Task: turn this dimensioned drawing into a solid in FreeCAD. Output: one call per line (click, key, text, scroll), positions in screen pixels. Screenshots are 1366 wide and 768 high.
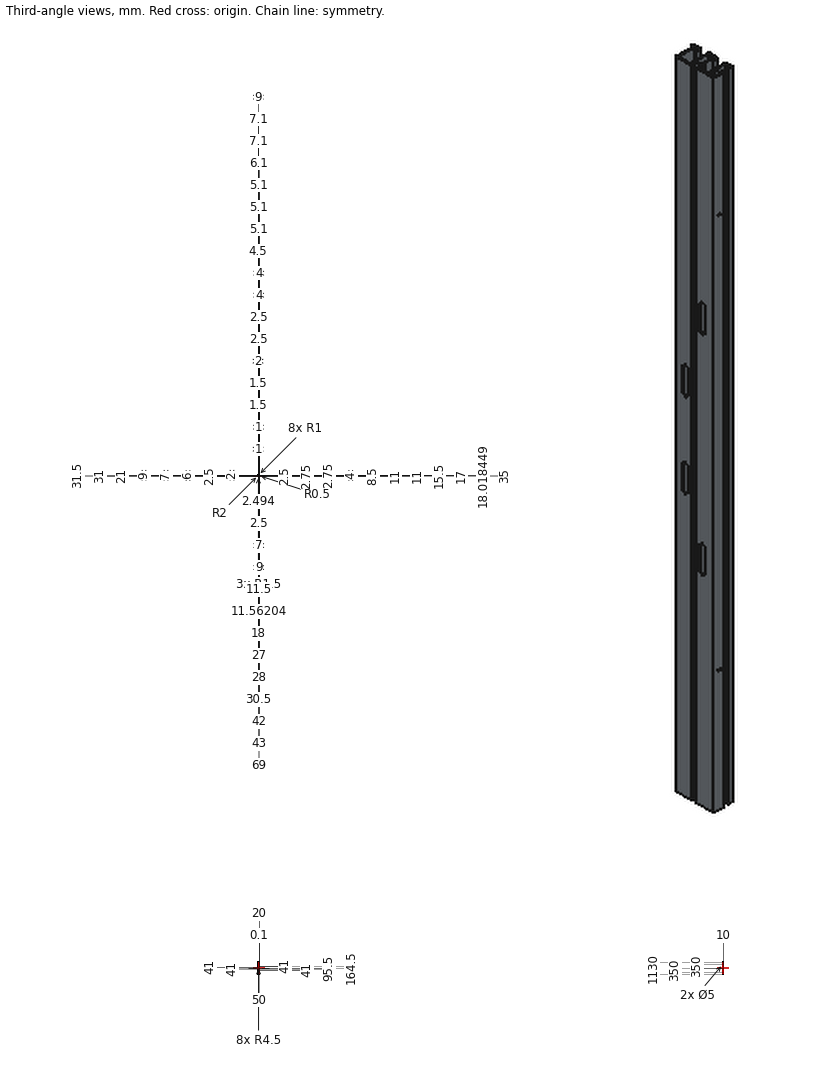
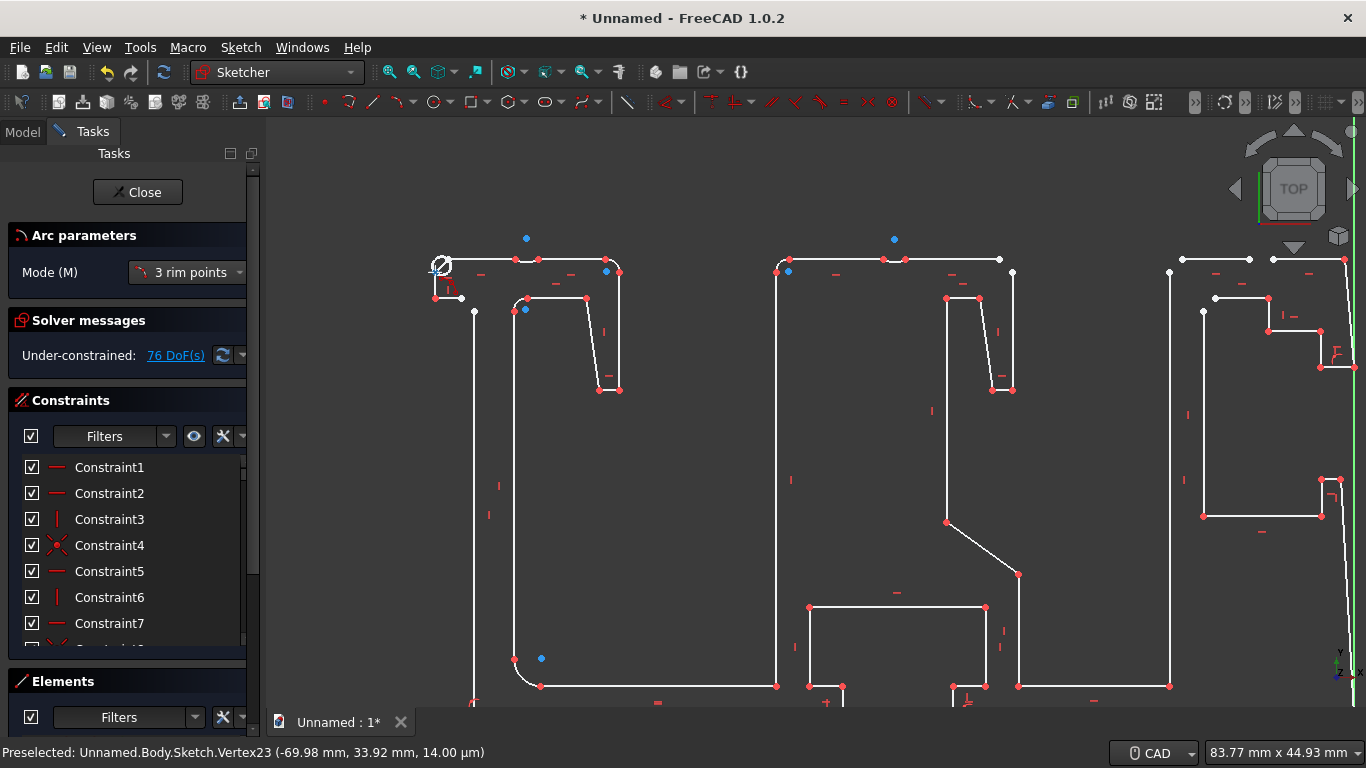
scroll(439, 262, up, 8)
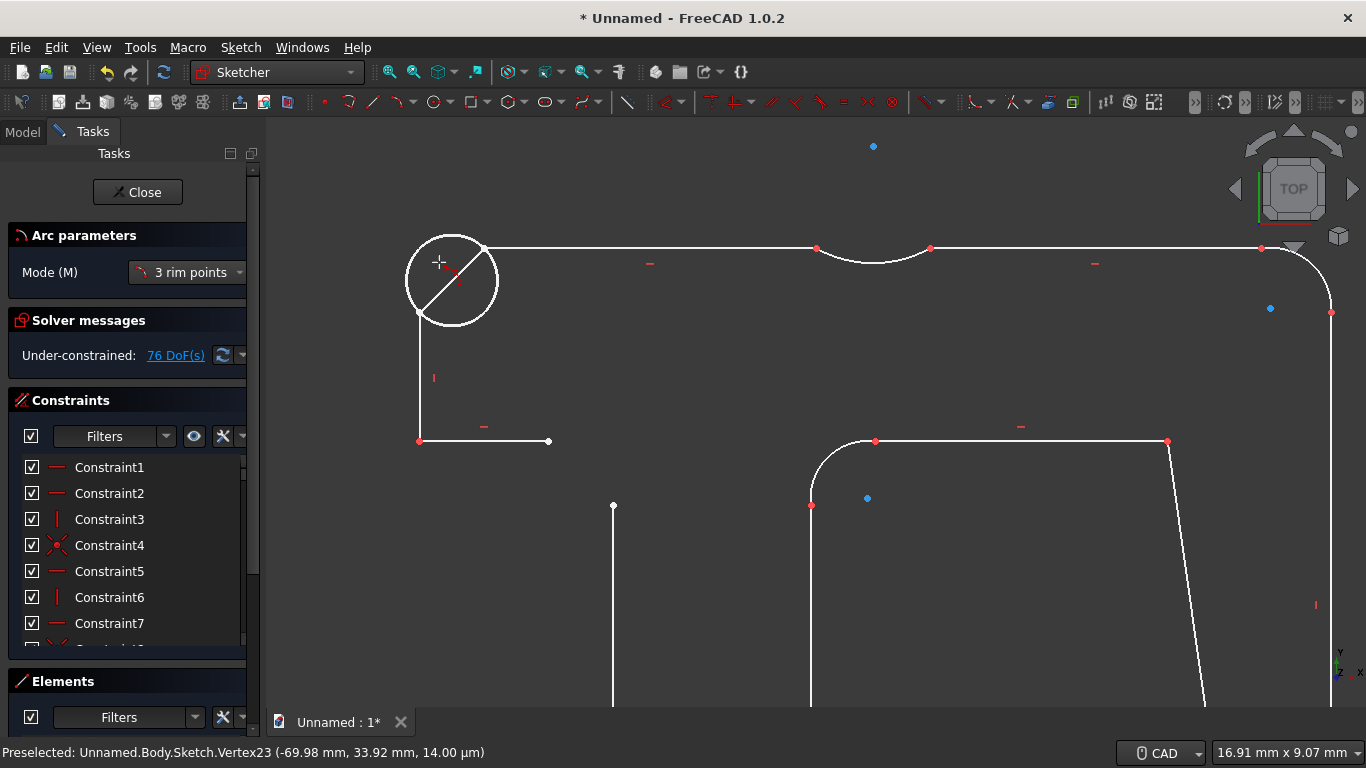
click(438, 261)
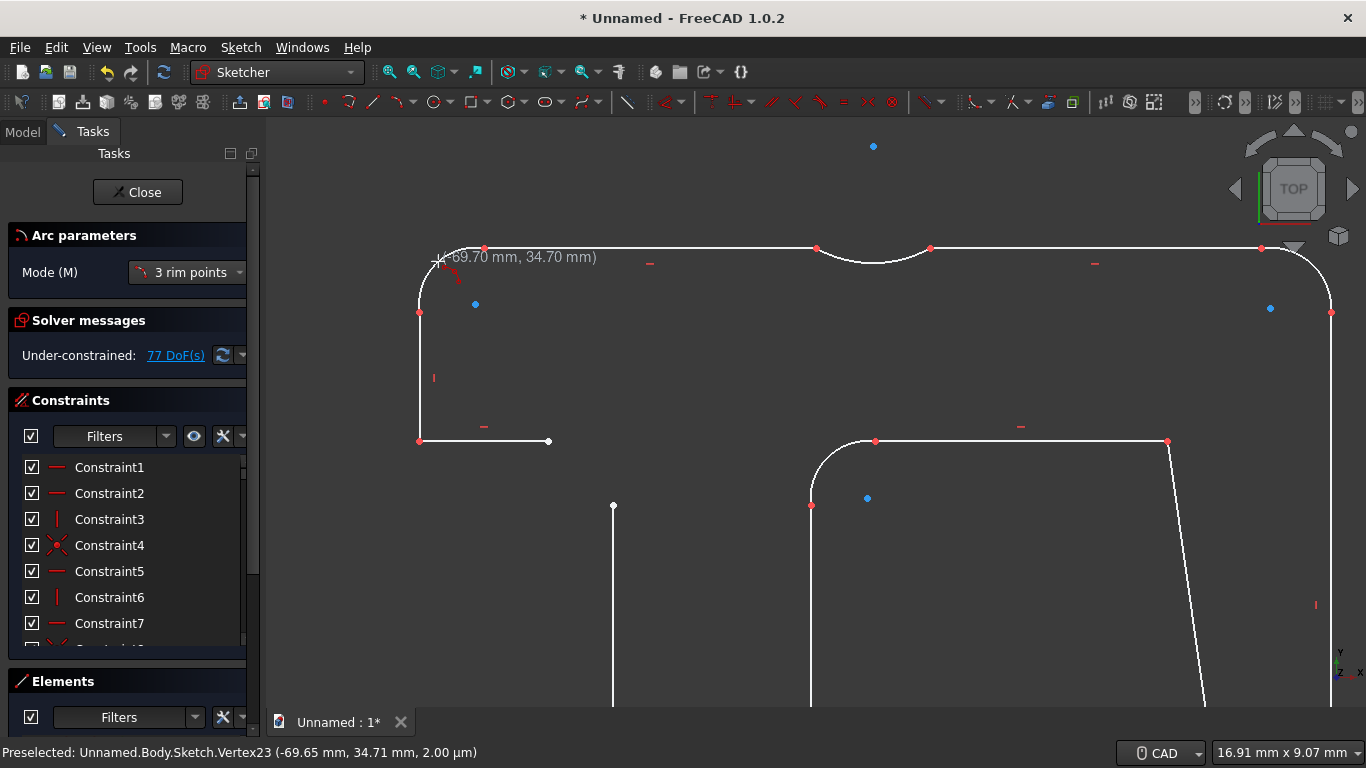
scroll(443, 260, down, 10)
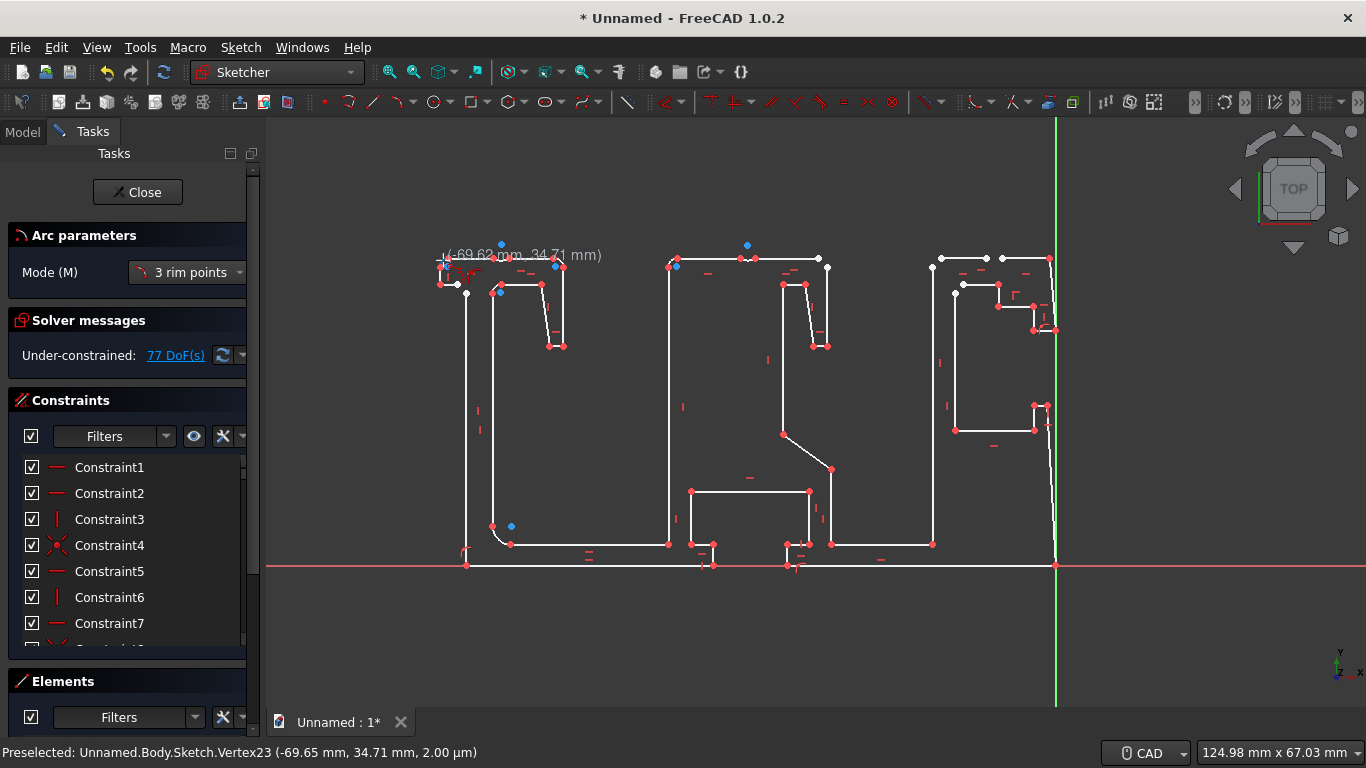
scroll(457, 284, up, 3)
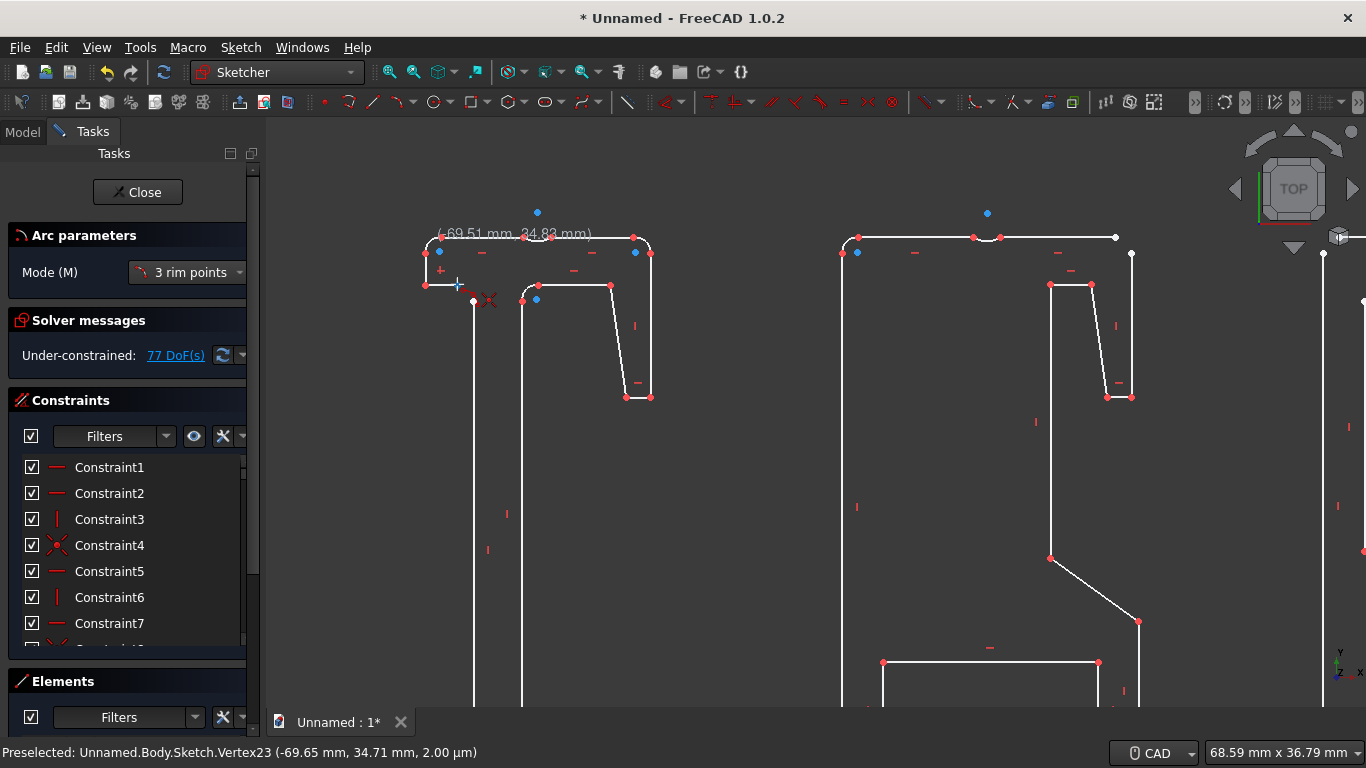
click(458, 285)
click(474, 301)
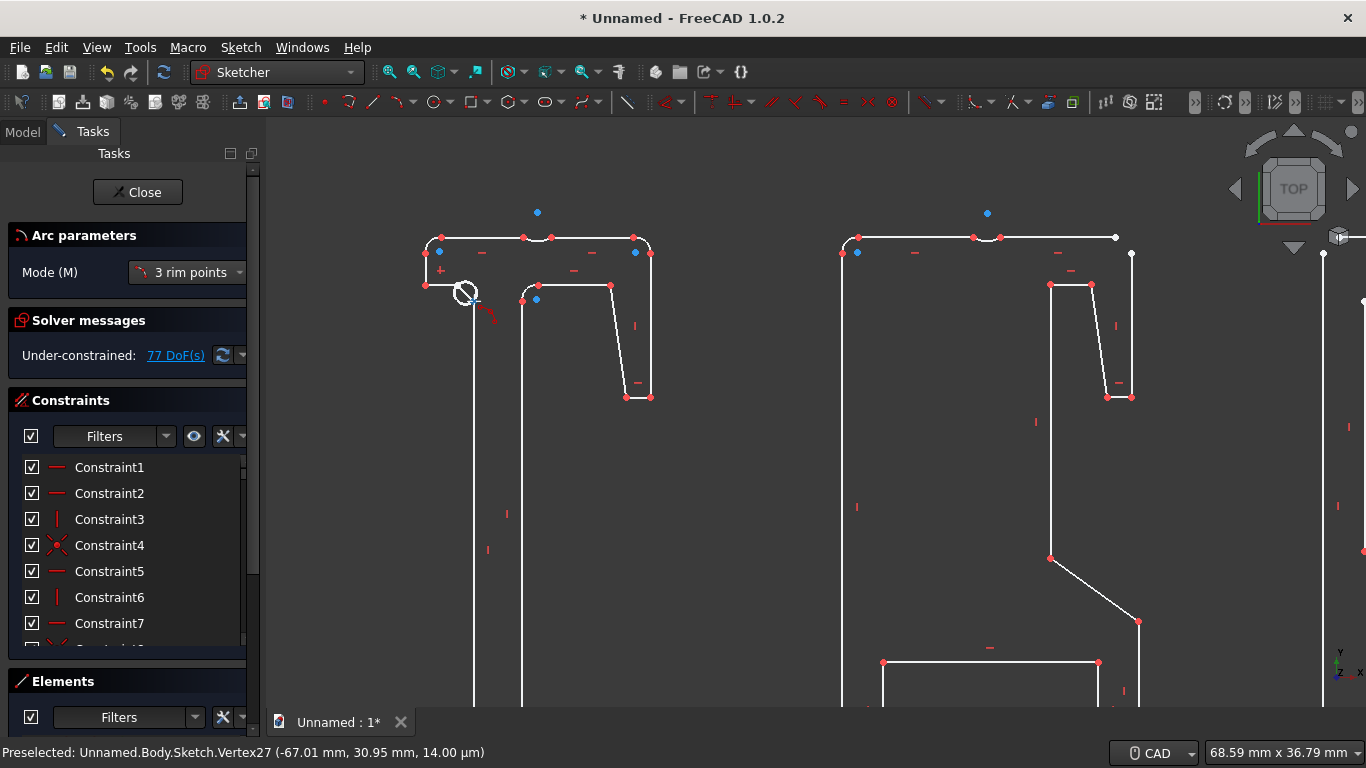
scroll(469, 289, up, 7)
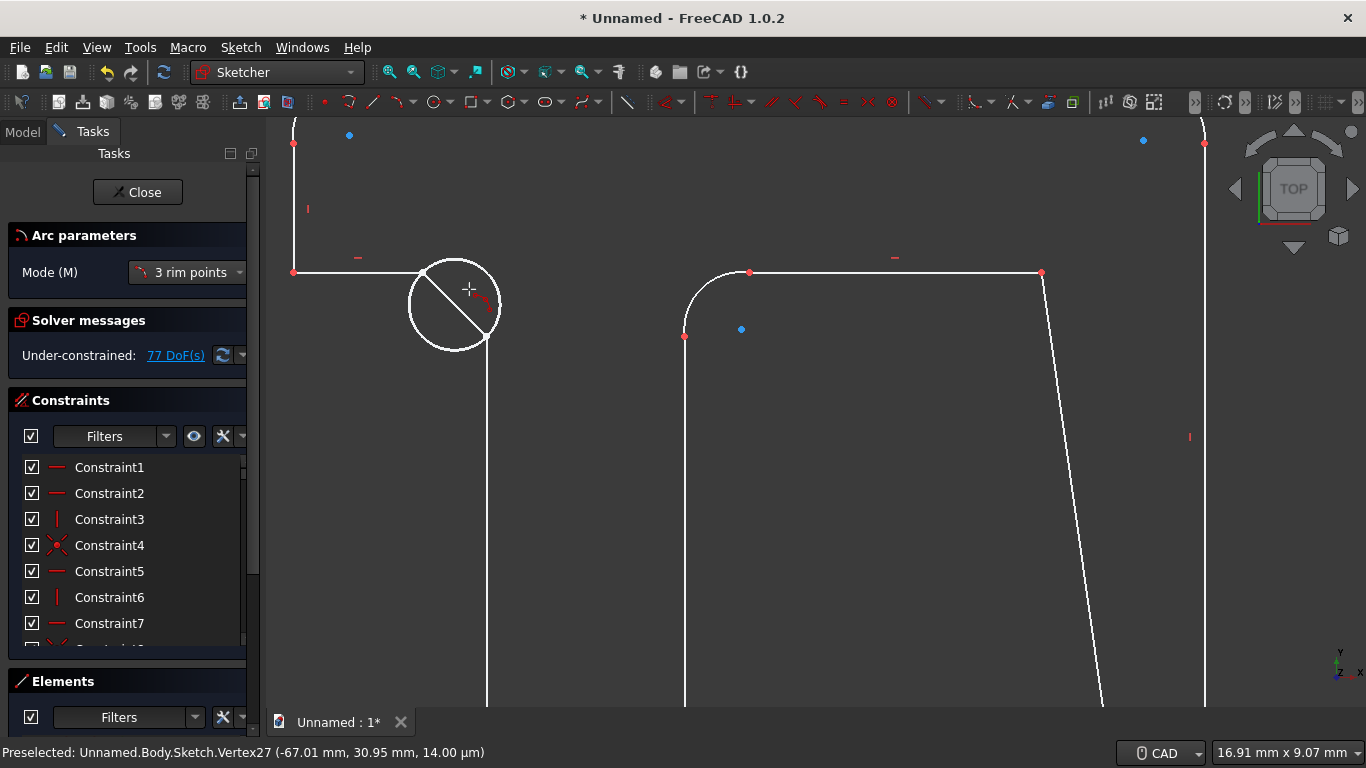
click(468, 288)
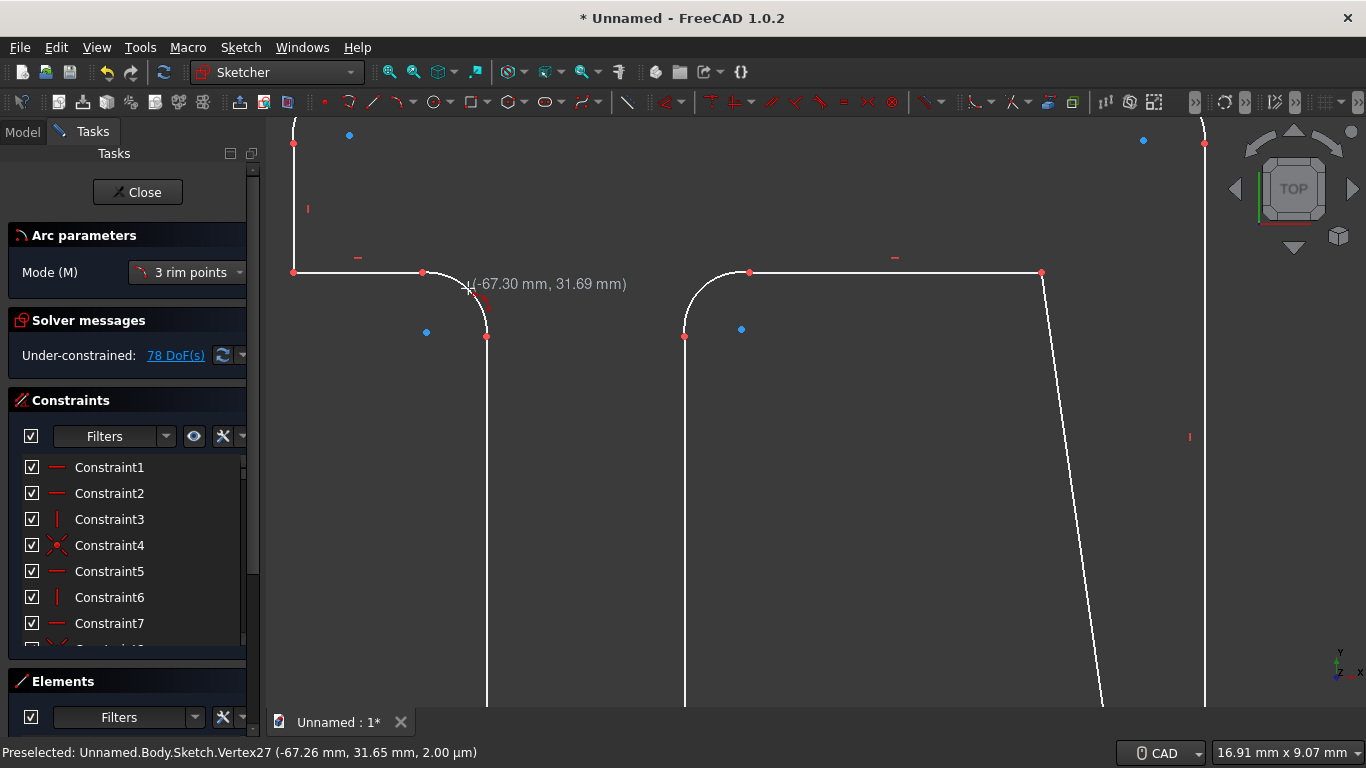
scroll(462, 287, down, 10)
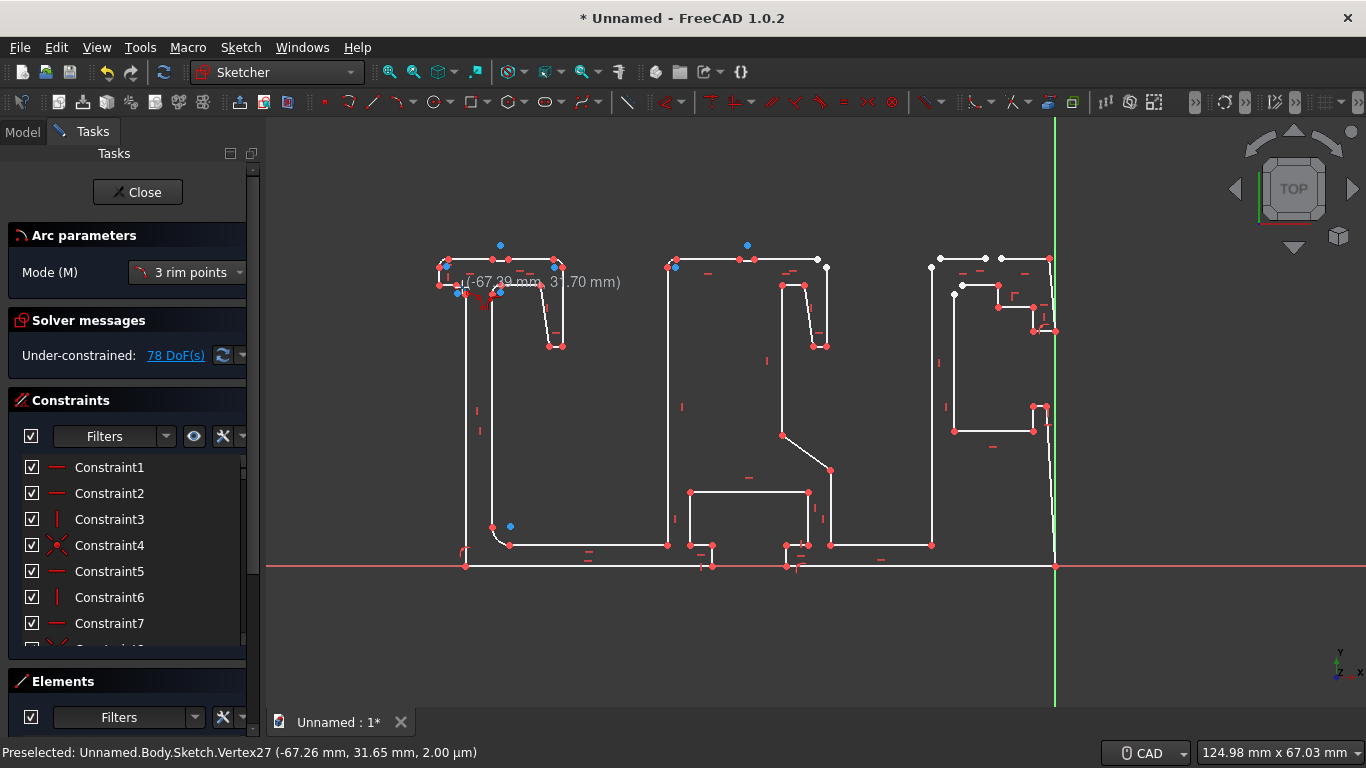
scroll(954, 294, up, 2)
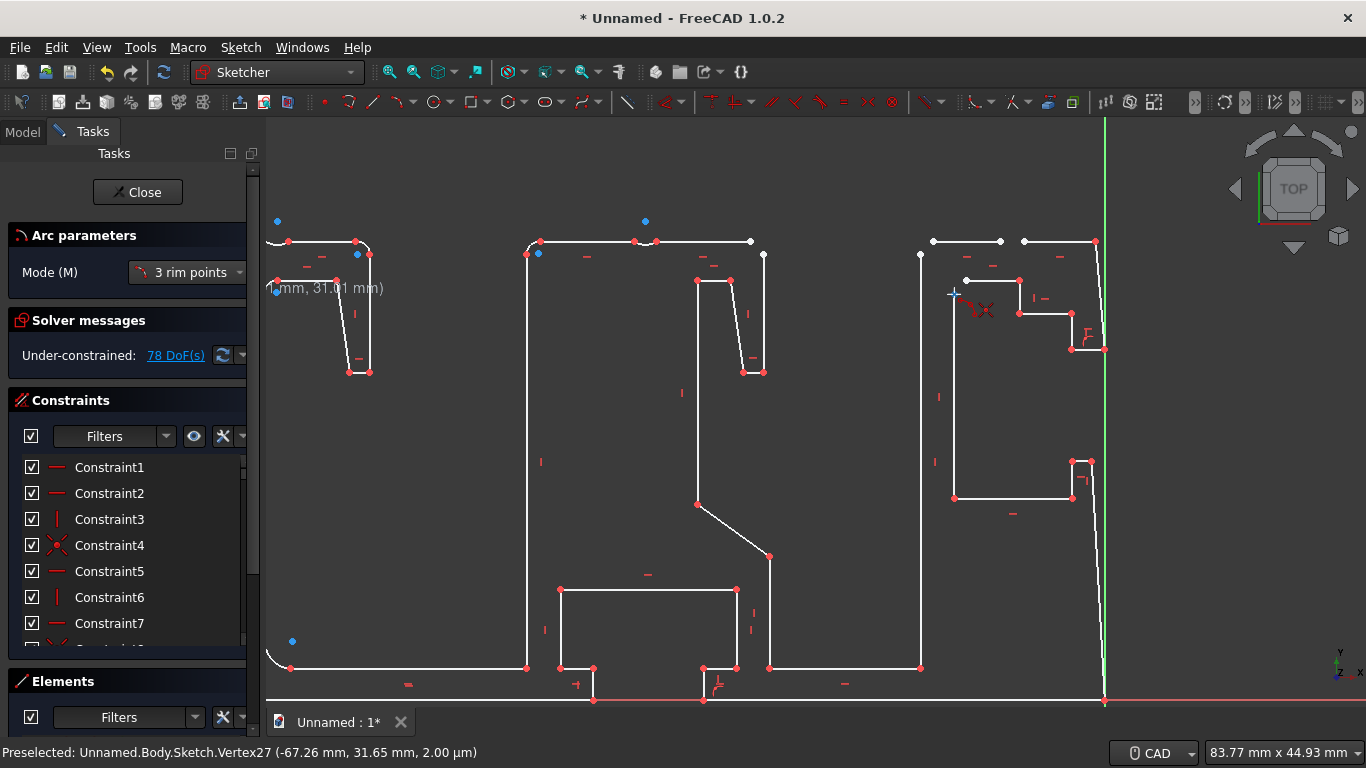
click(954, 294)
click(967, 281)